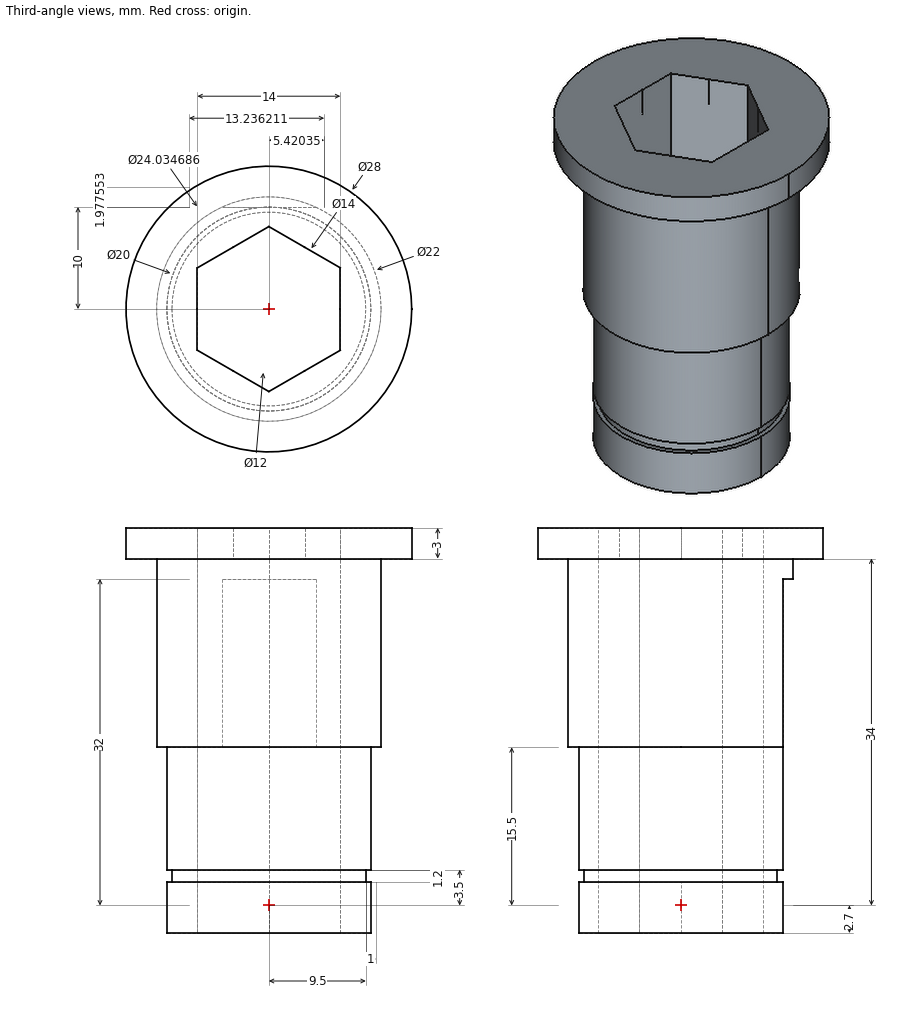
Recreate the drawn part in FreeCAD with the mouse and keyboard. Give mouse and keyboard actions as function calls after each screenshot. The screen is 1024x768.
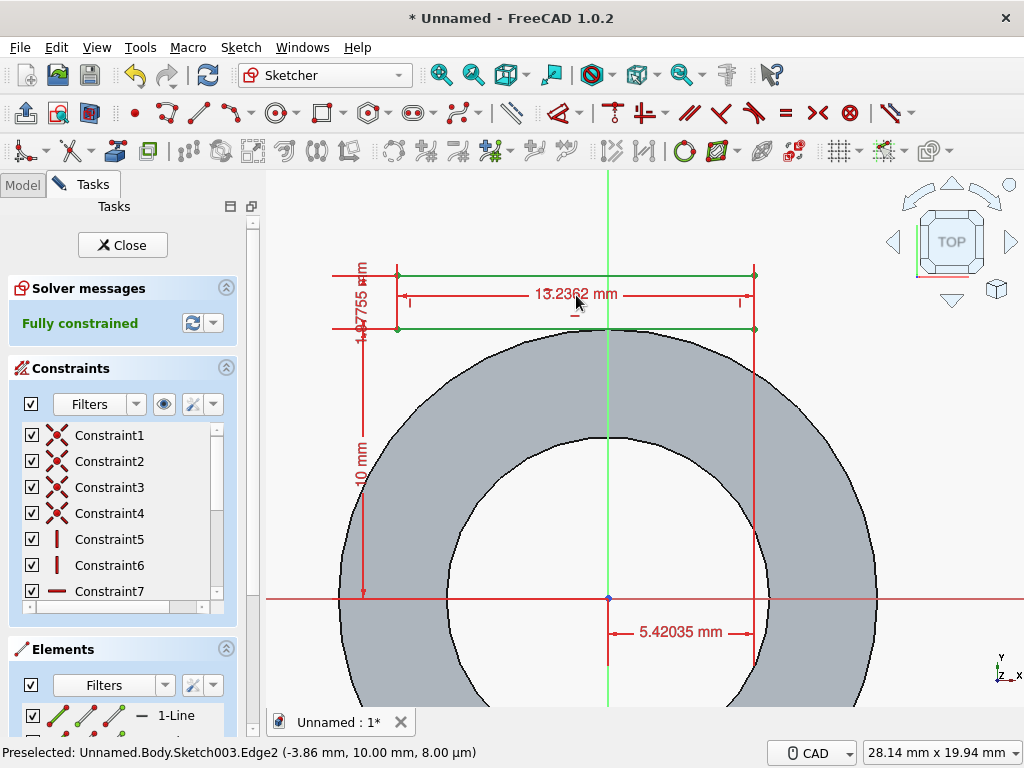
click(123, 245)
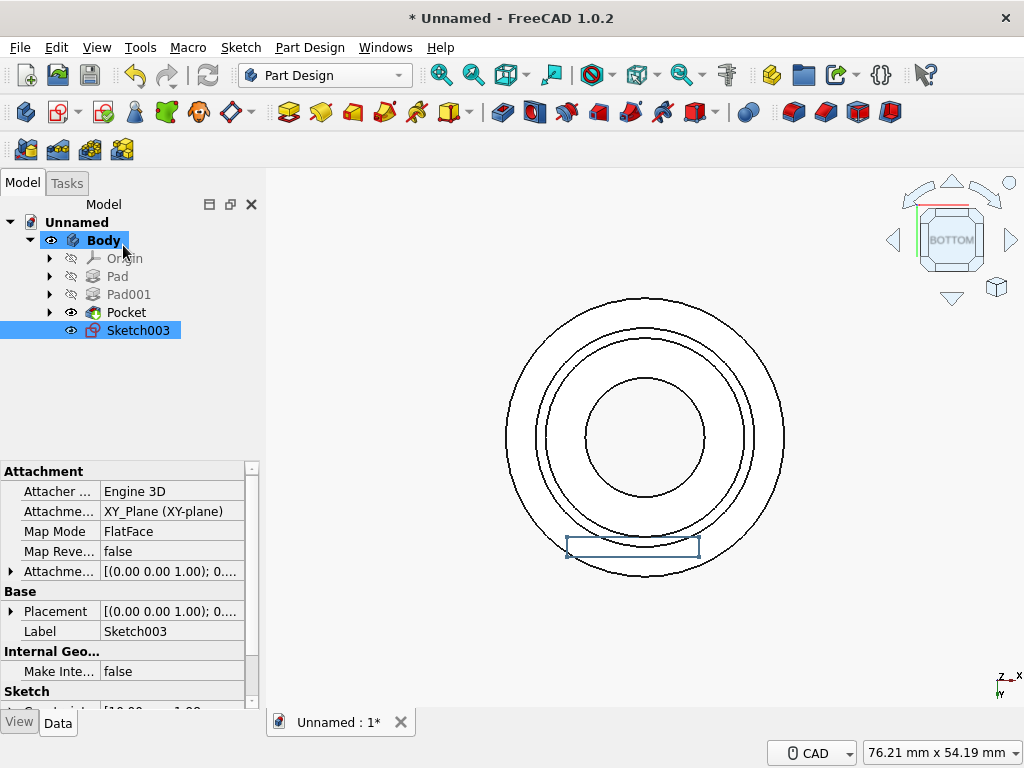
click(504, 112)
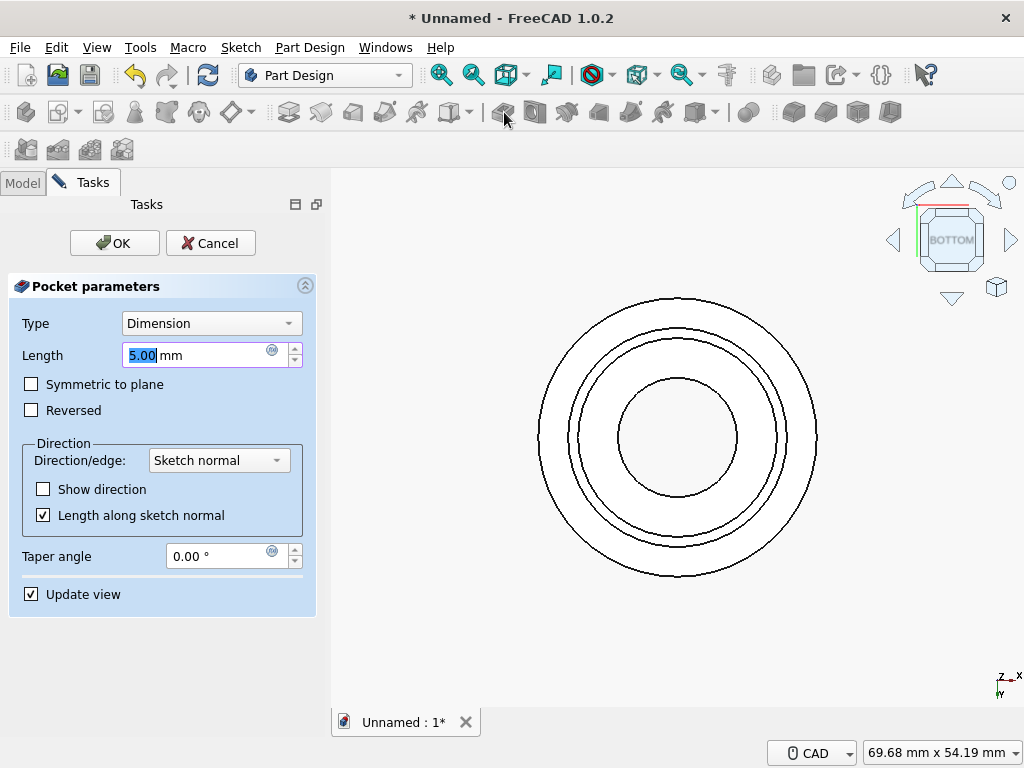
text(32)
key(Tab)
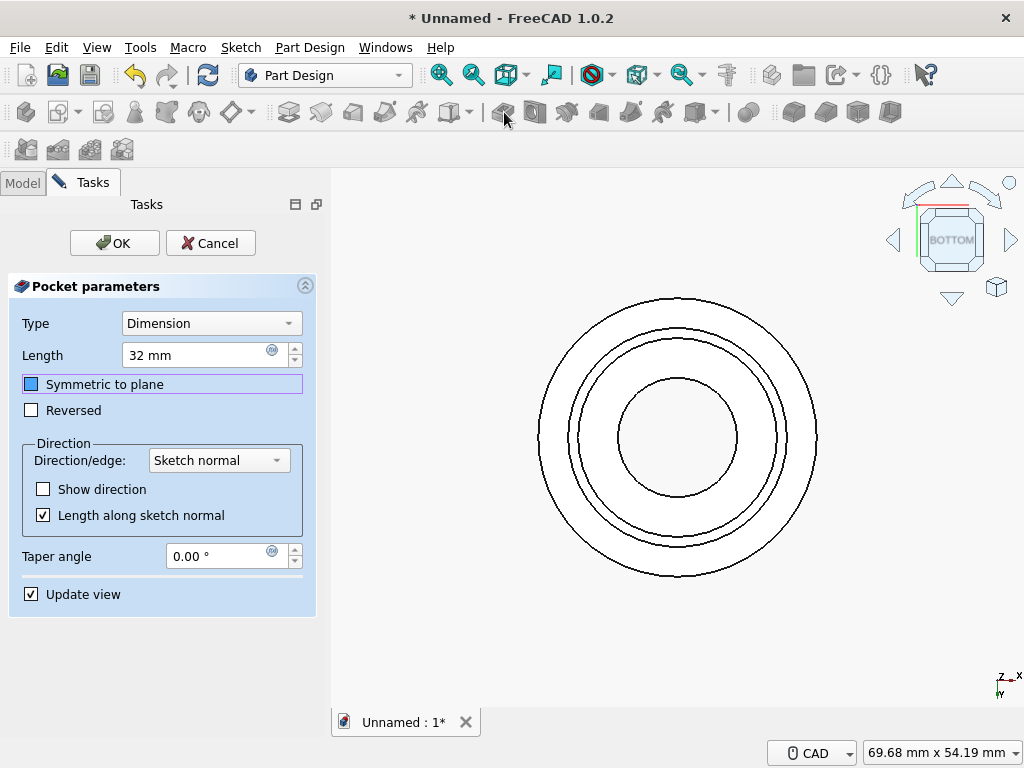
click(30, 410)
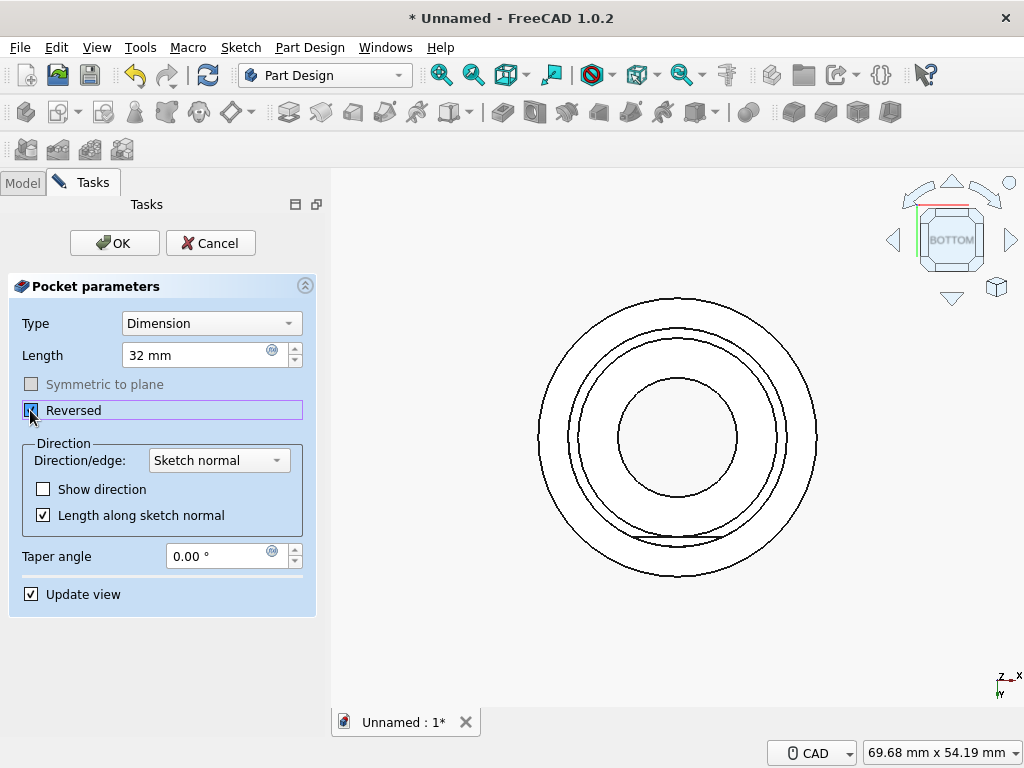
click(115, 243)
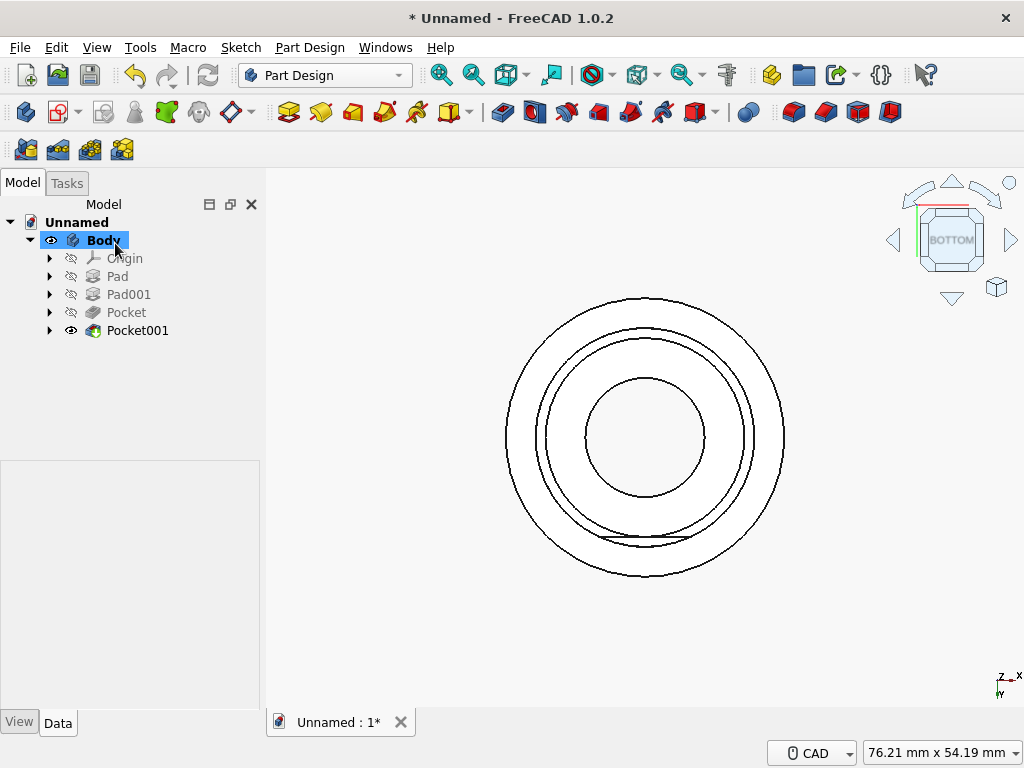
key(0)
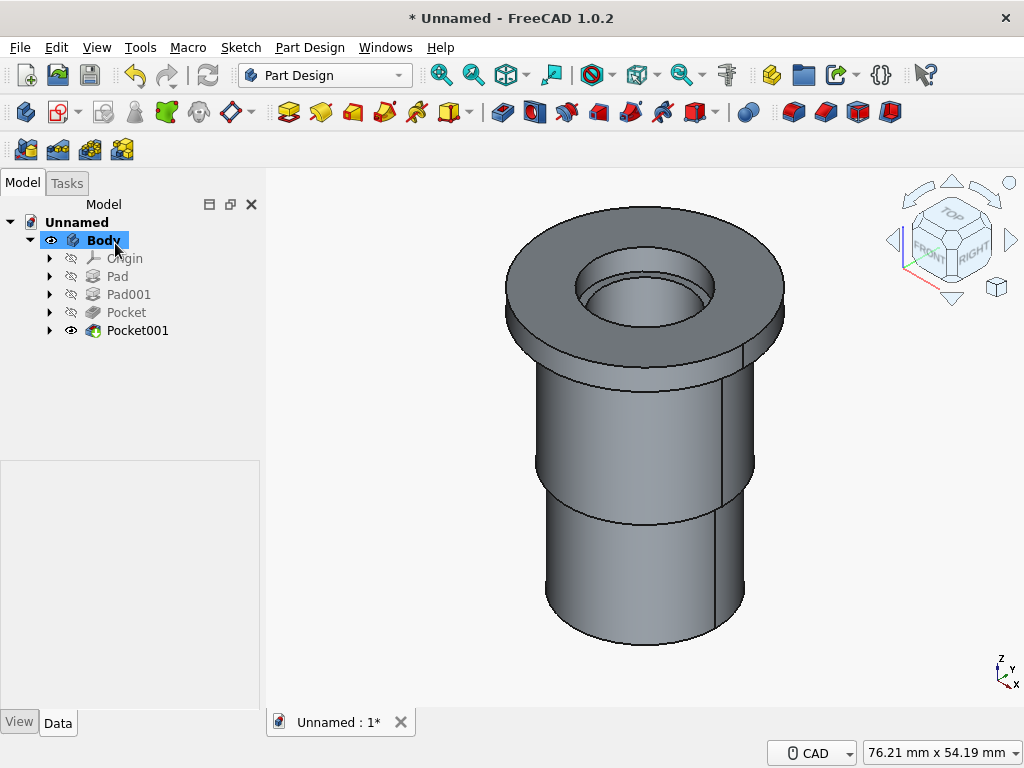
click(645, 351)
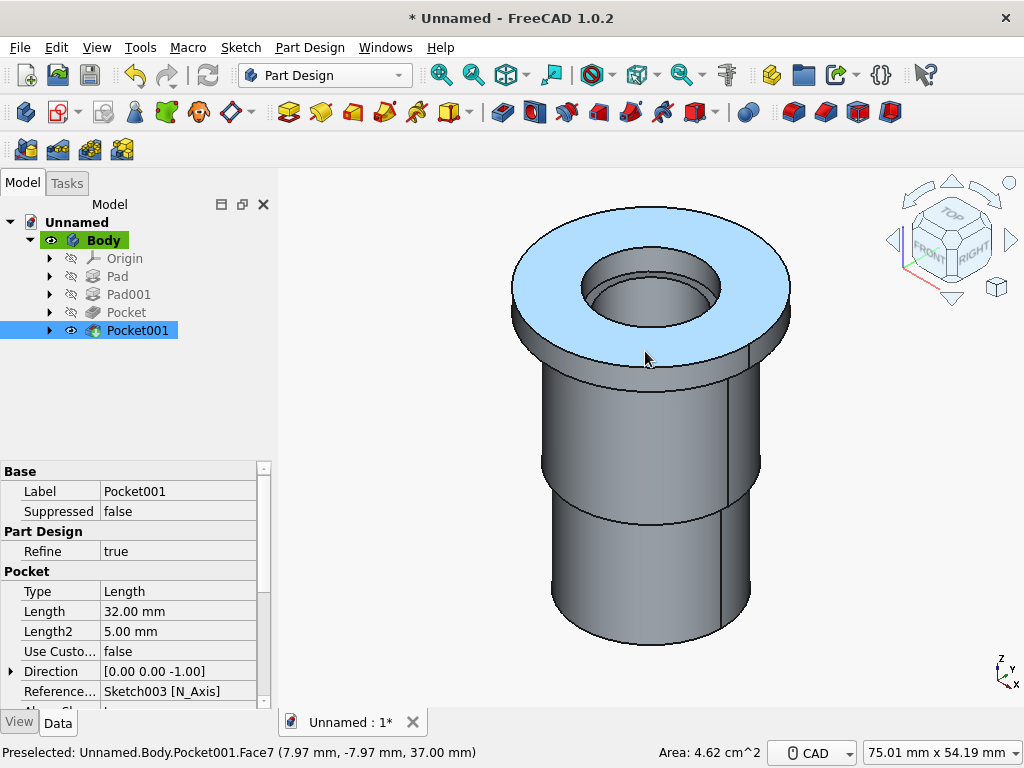
click(58, 112)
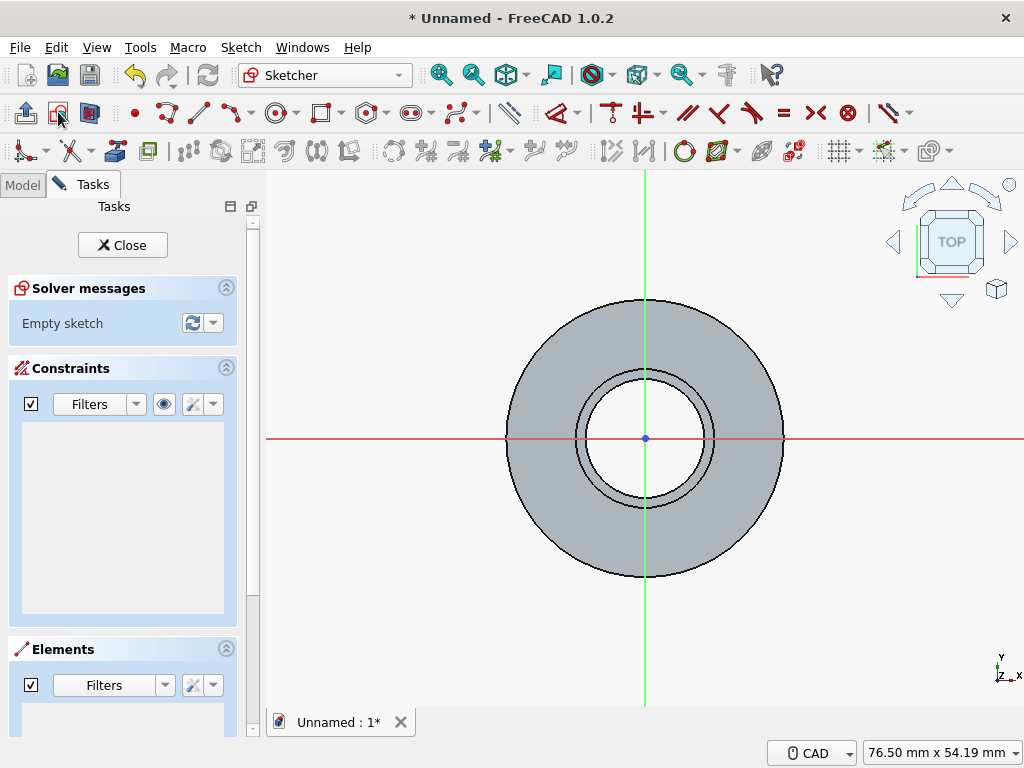
scroll(701, 438, up, 4)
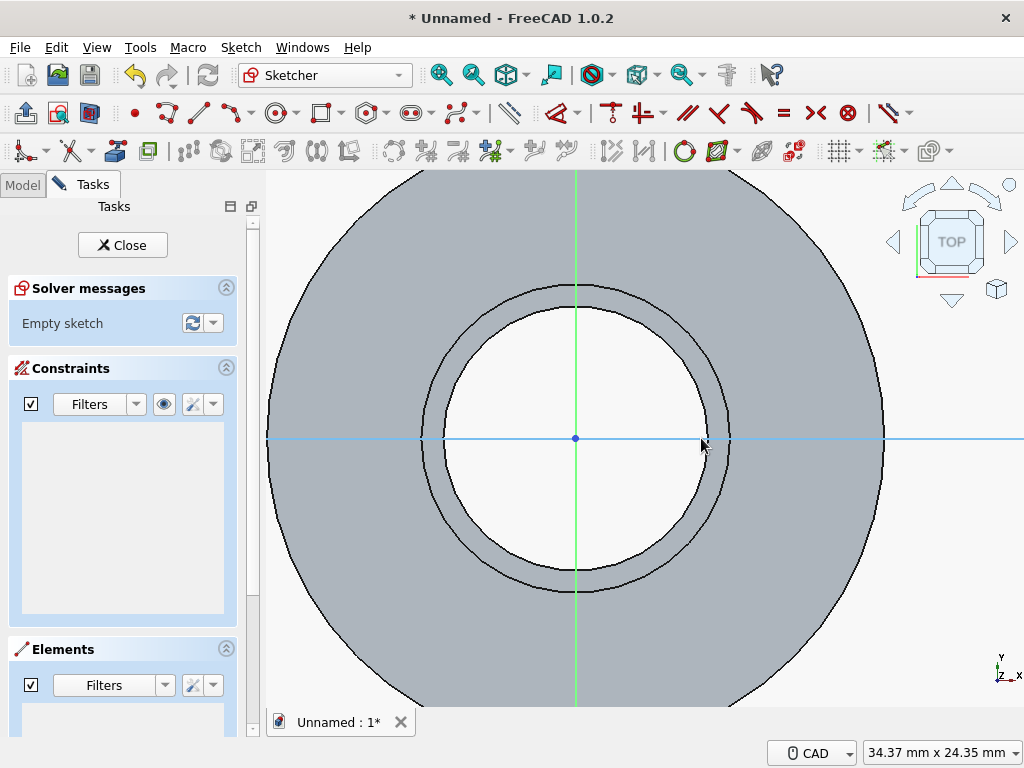
click(366, 114)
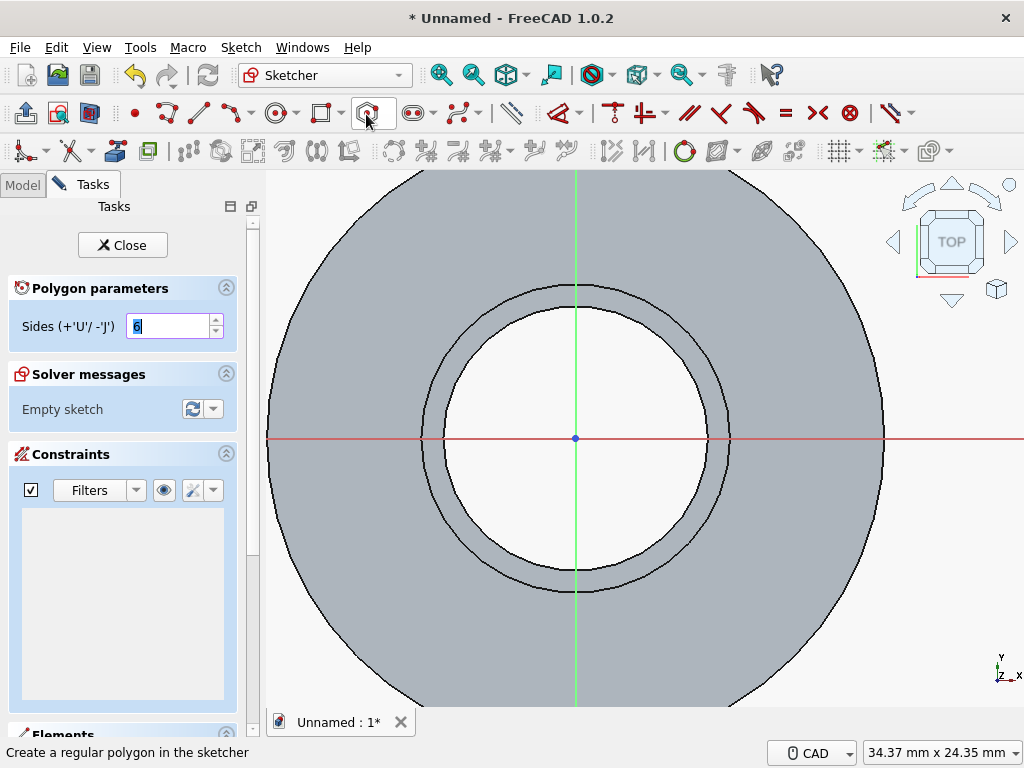
click(576, 438)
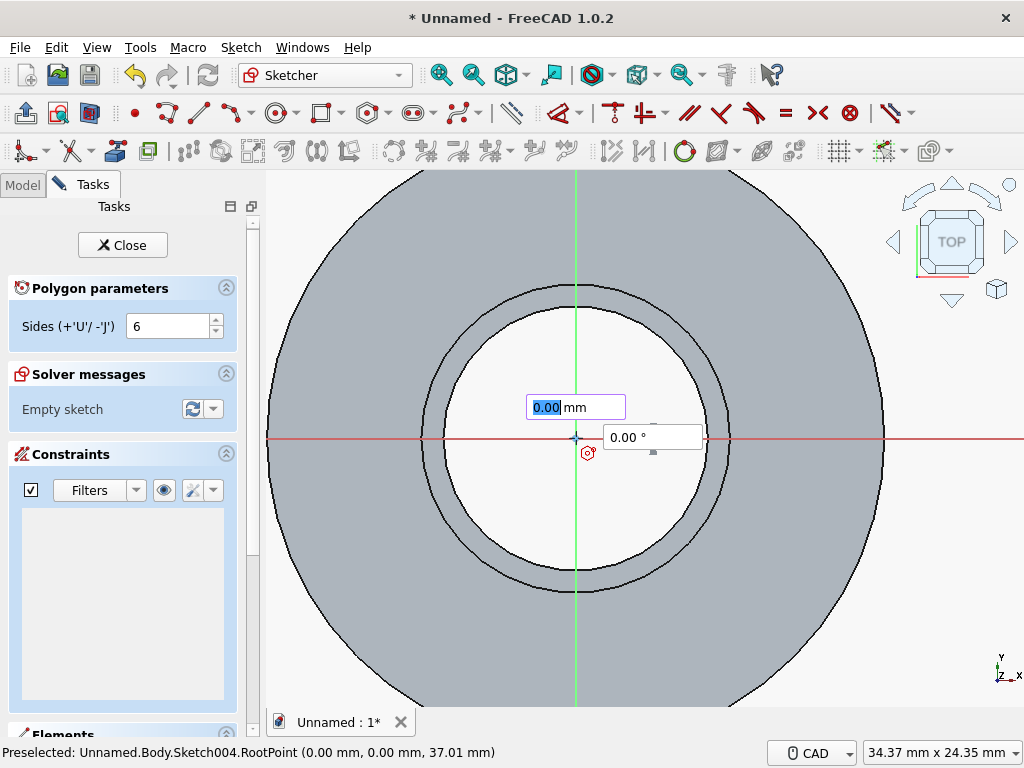
click(576, 260)
right_click(576, 260)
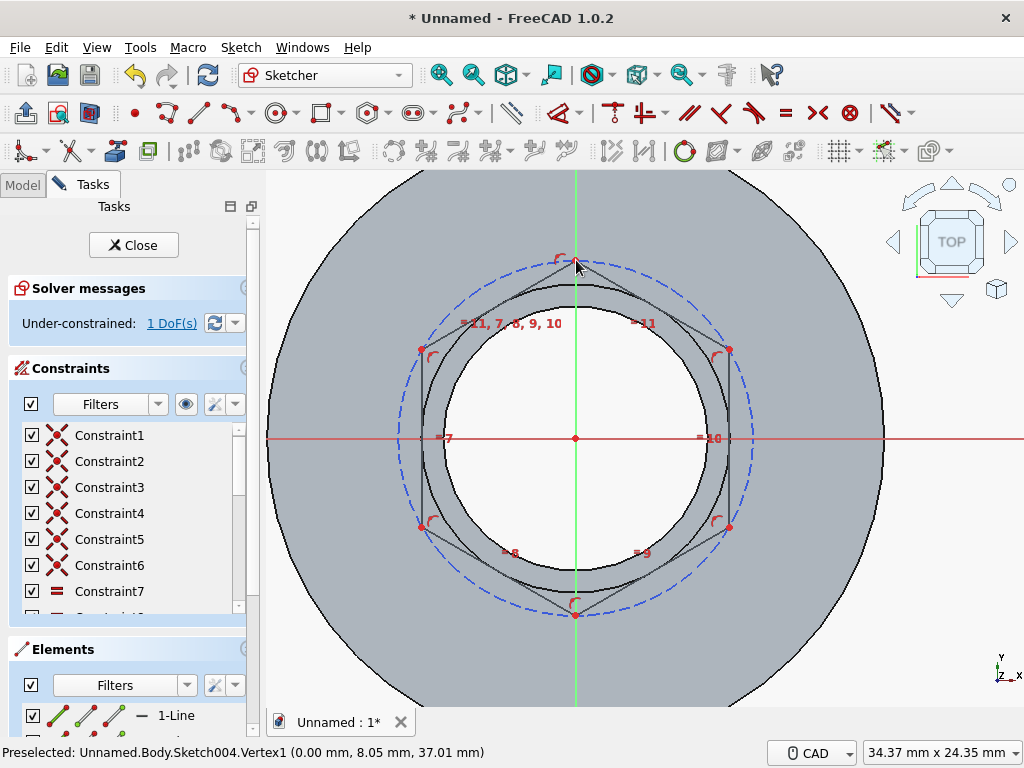
click(558, 114)